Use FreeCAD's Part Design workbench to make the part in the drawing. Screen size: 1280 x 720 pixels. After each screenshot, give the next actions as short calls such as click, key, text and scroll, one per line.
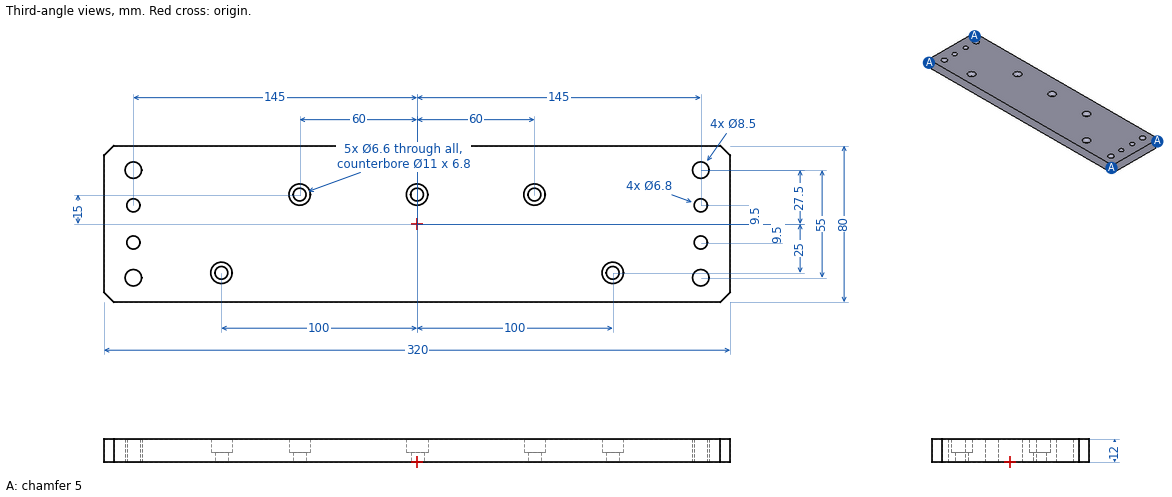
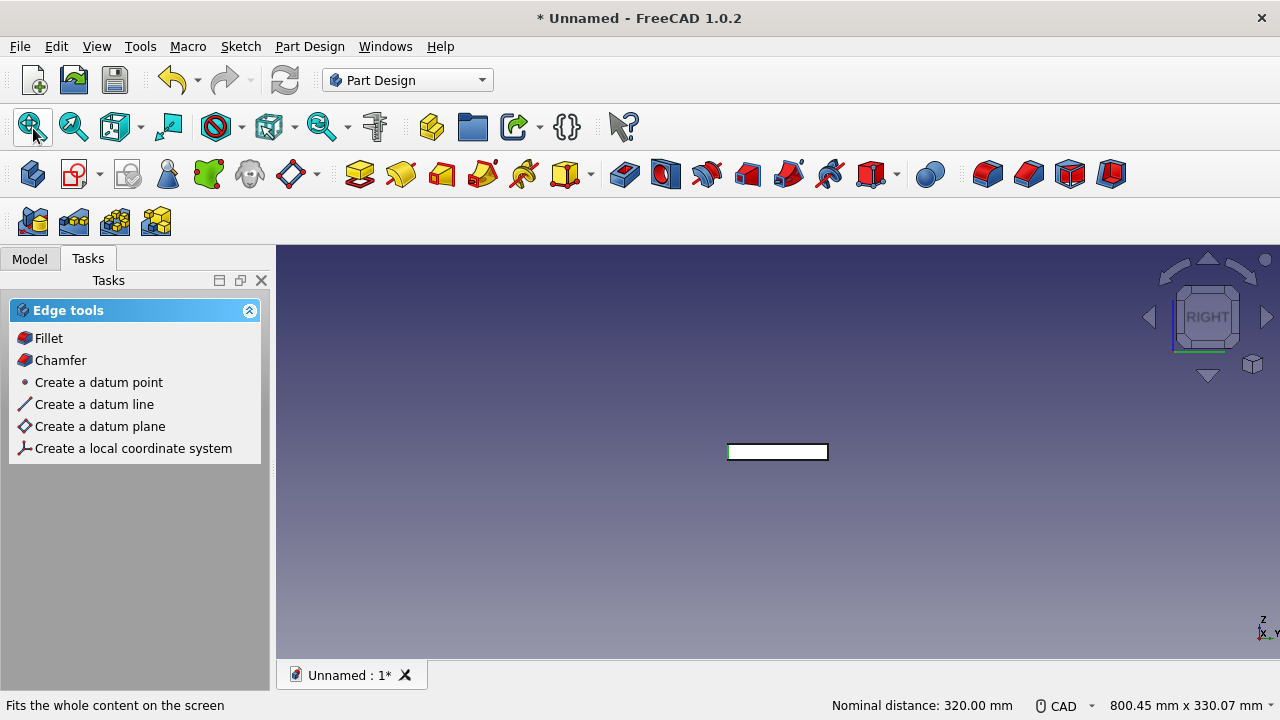
key(v)
key(f)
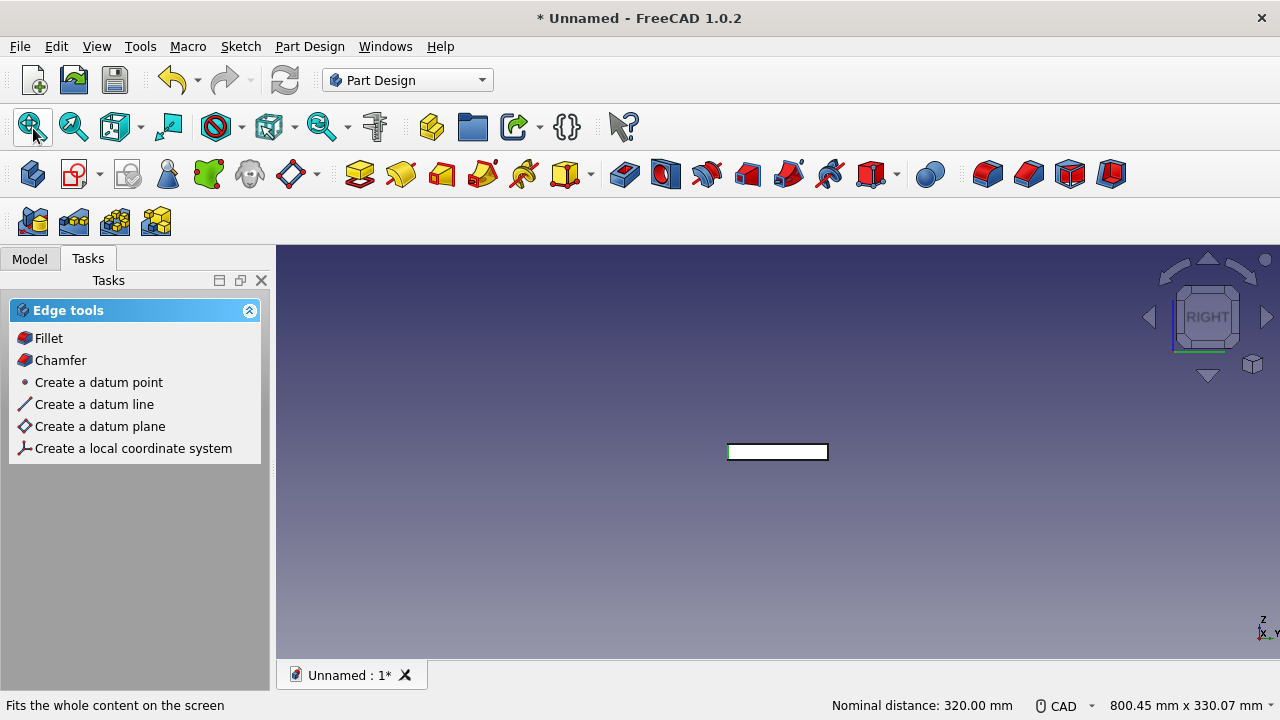
click(828, 451, ctrl)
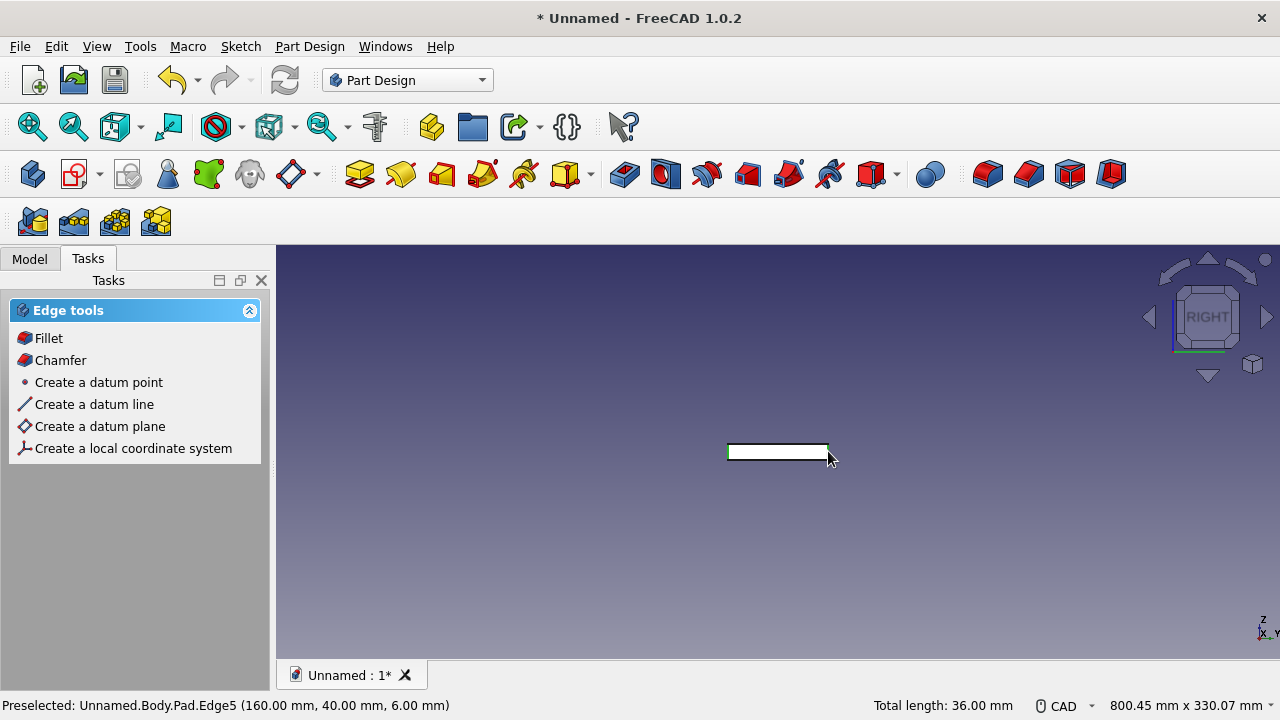
scroll(828, 451, up, 5)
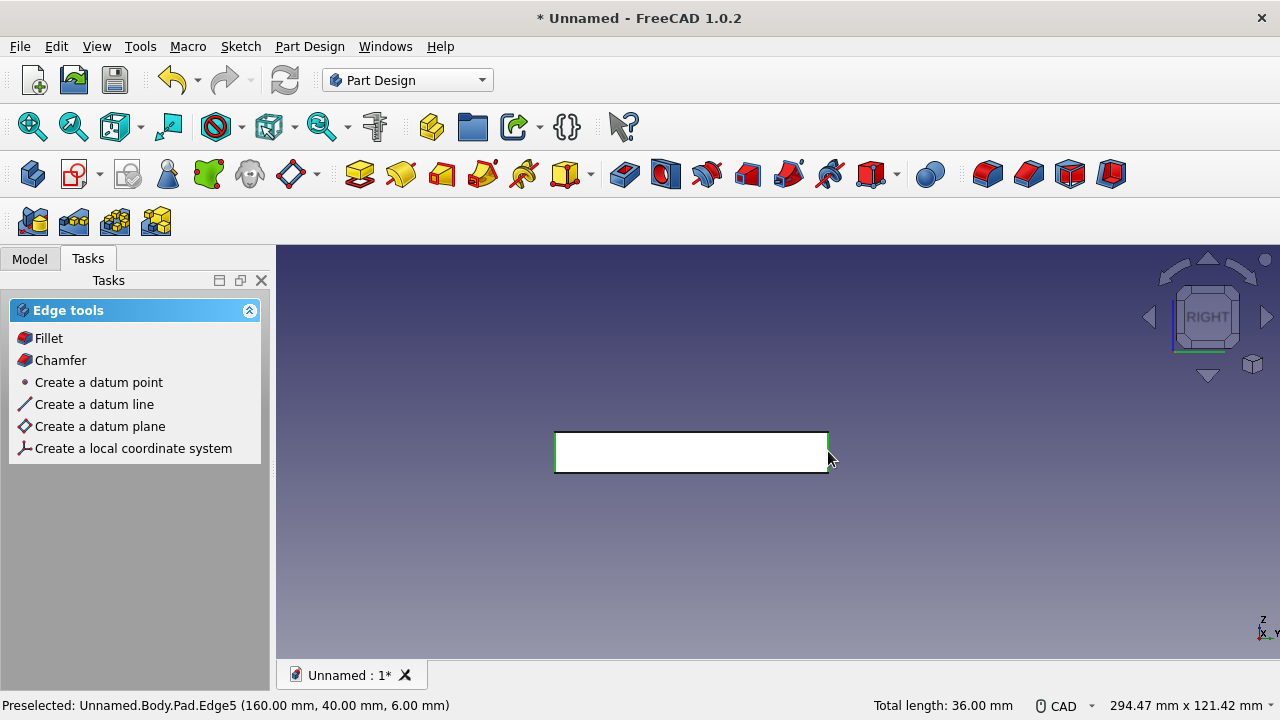
click(33, 128)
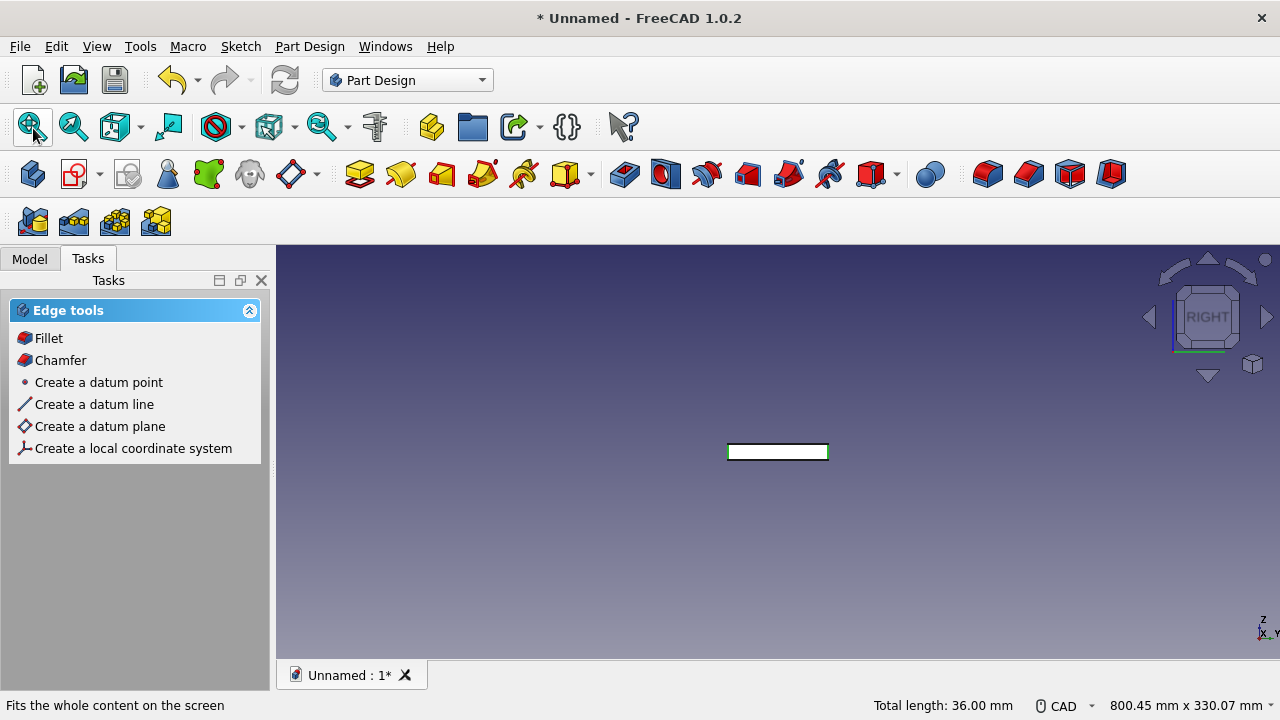
key(5)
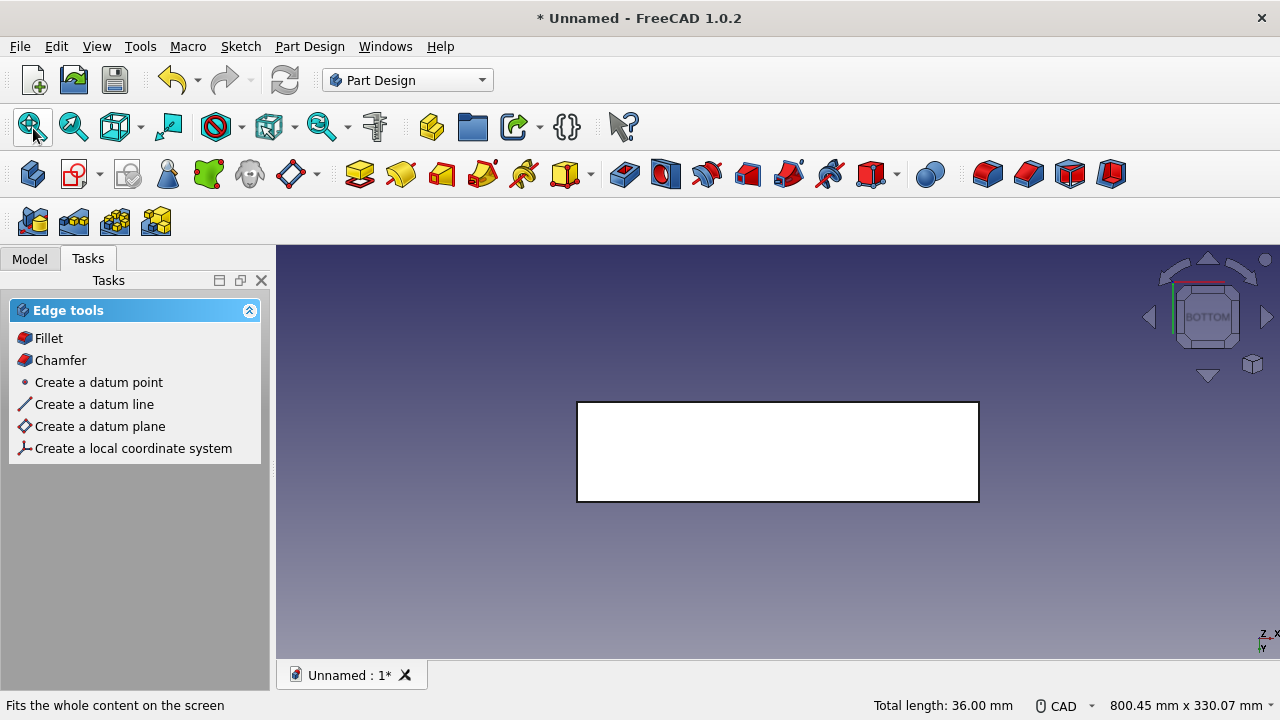
click(33, 128)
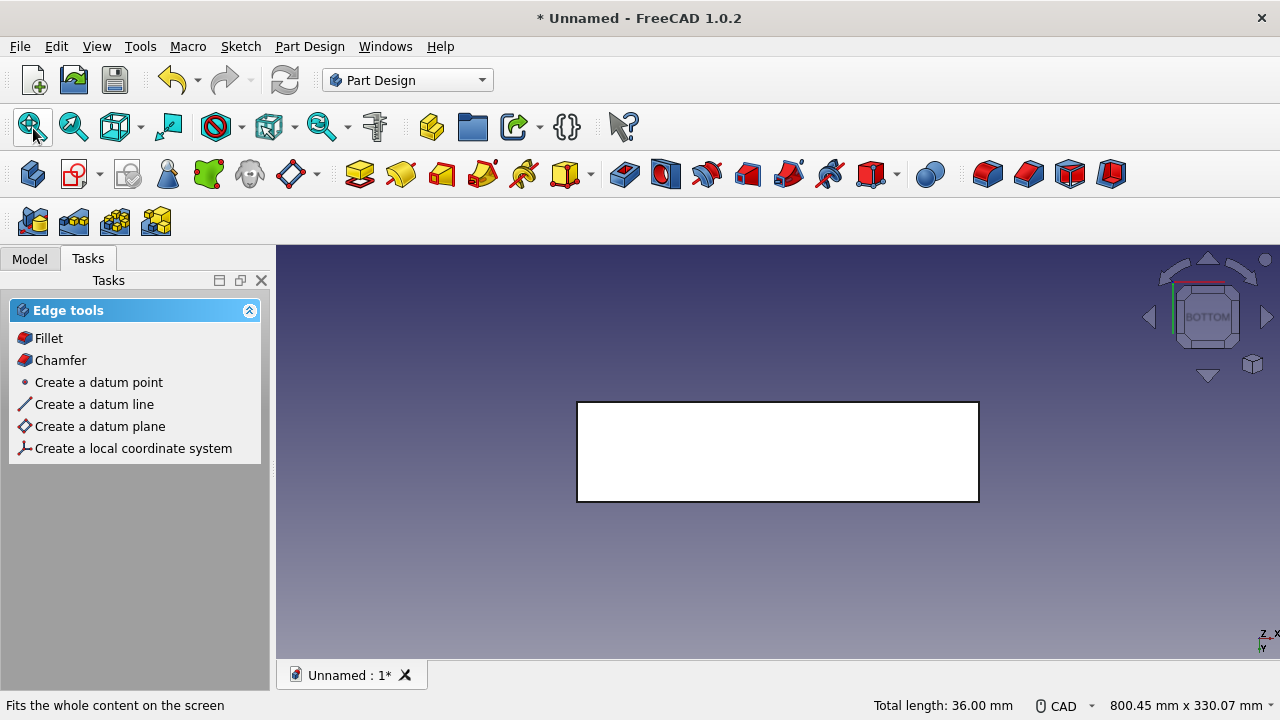
scroll(577, 501, up, 5)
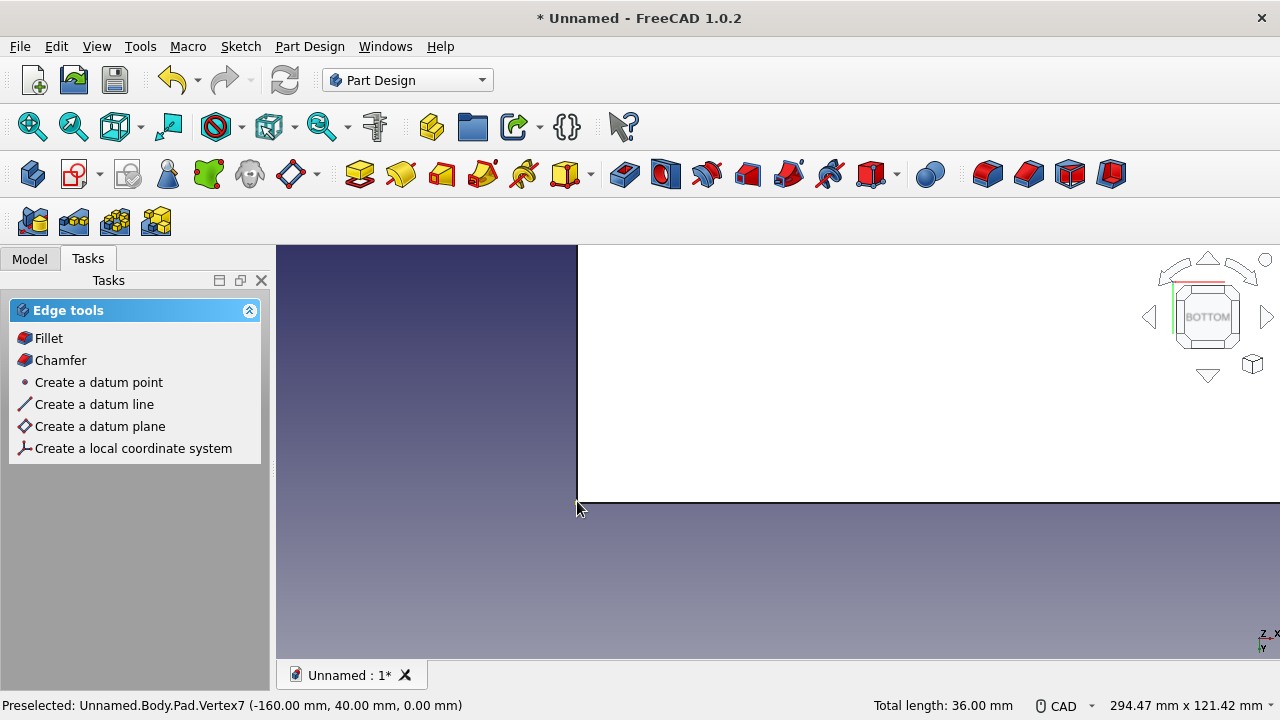
click(33, 128)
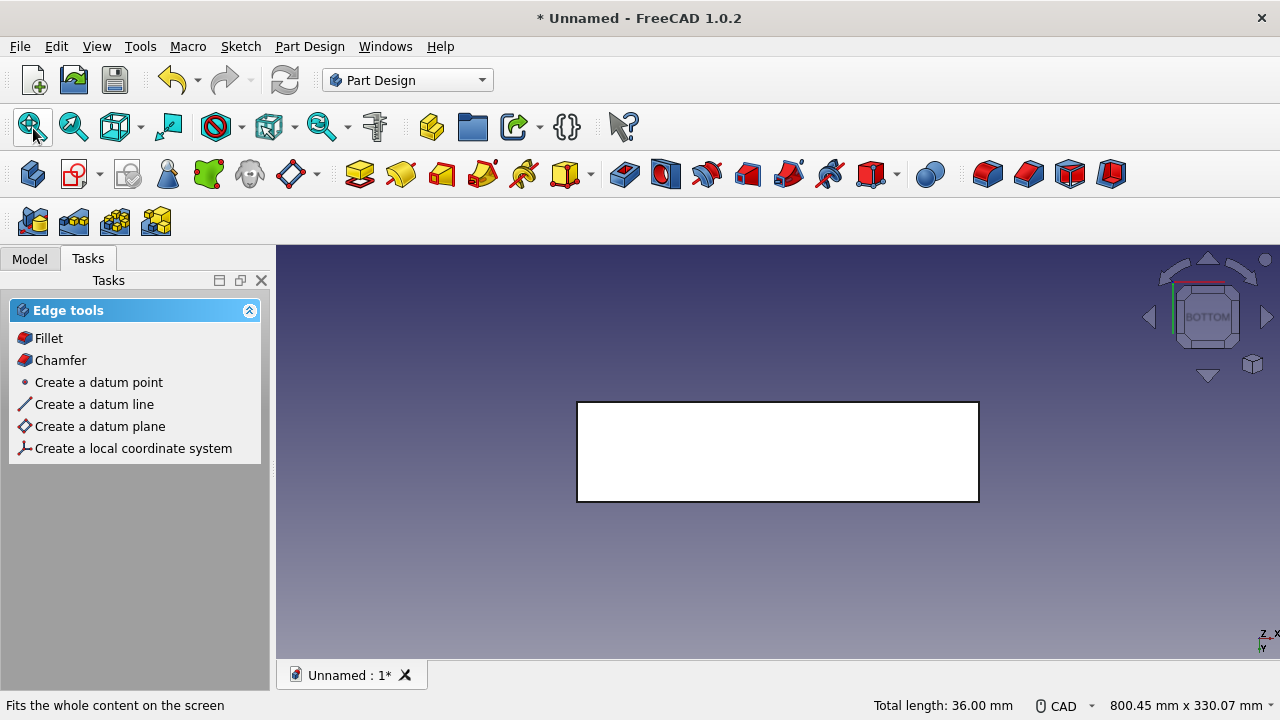
key(4)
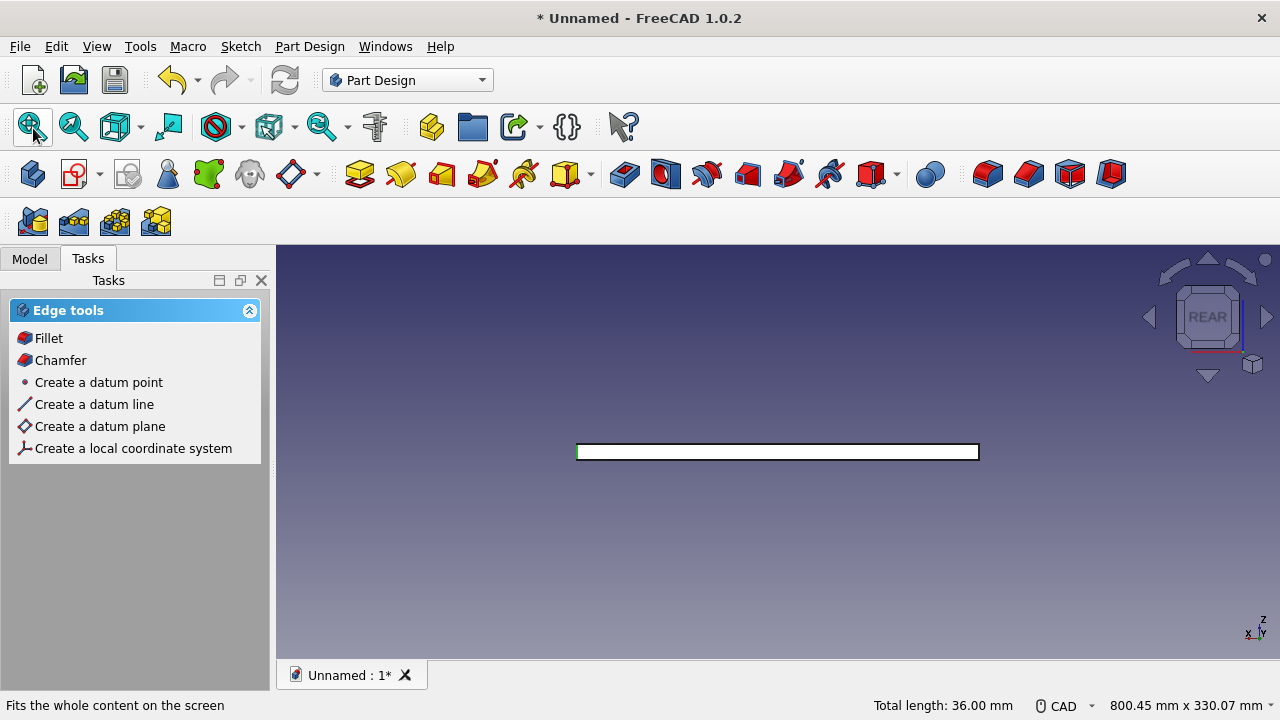
click(33, 128)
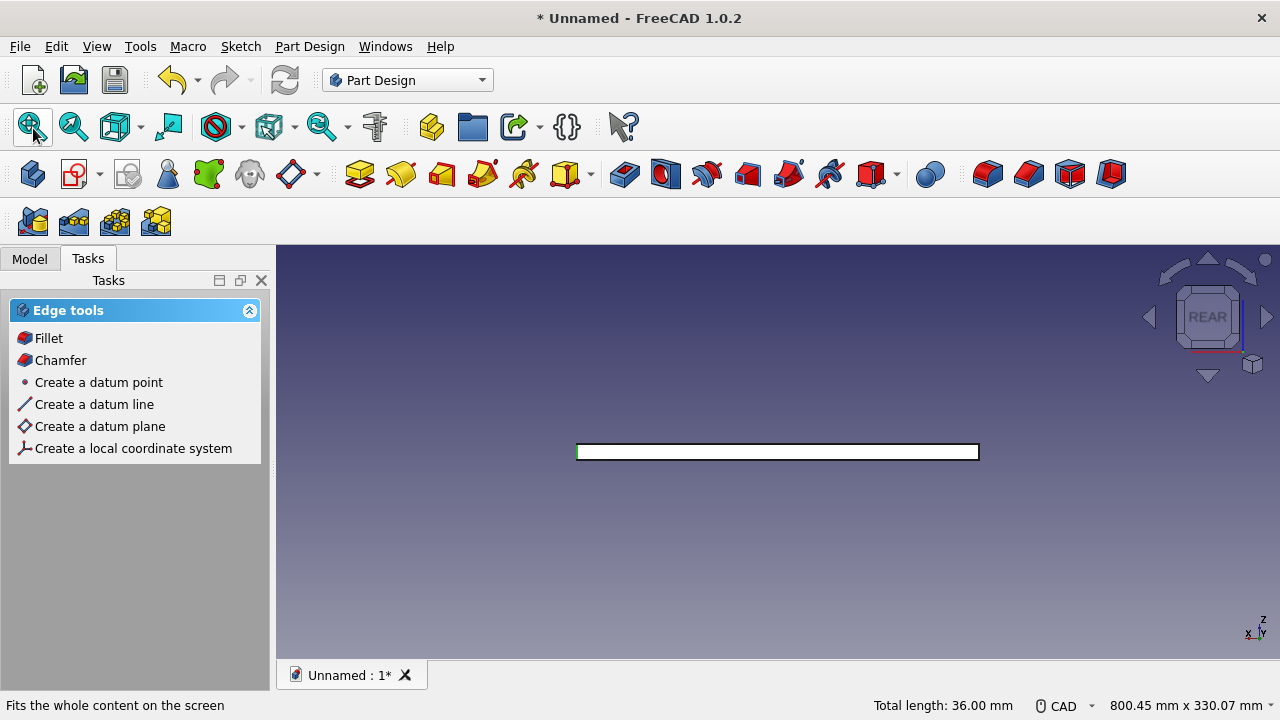
click(979, 451, ctrl)